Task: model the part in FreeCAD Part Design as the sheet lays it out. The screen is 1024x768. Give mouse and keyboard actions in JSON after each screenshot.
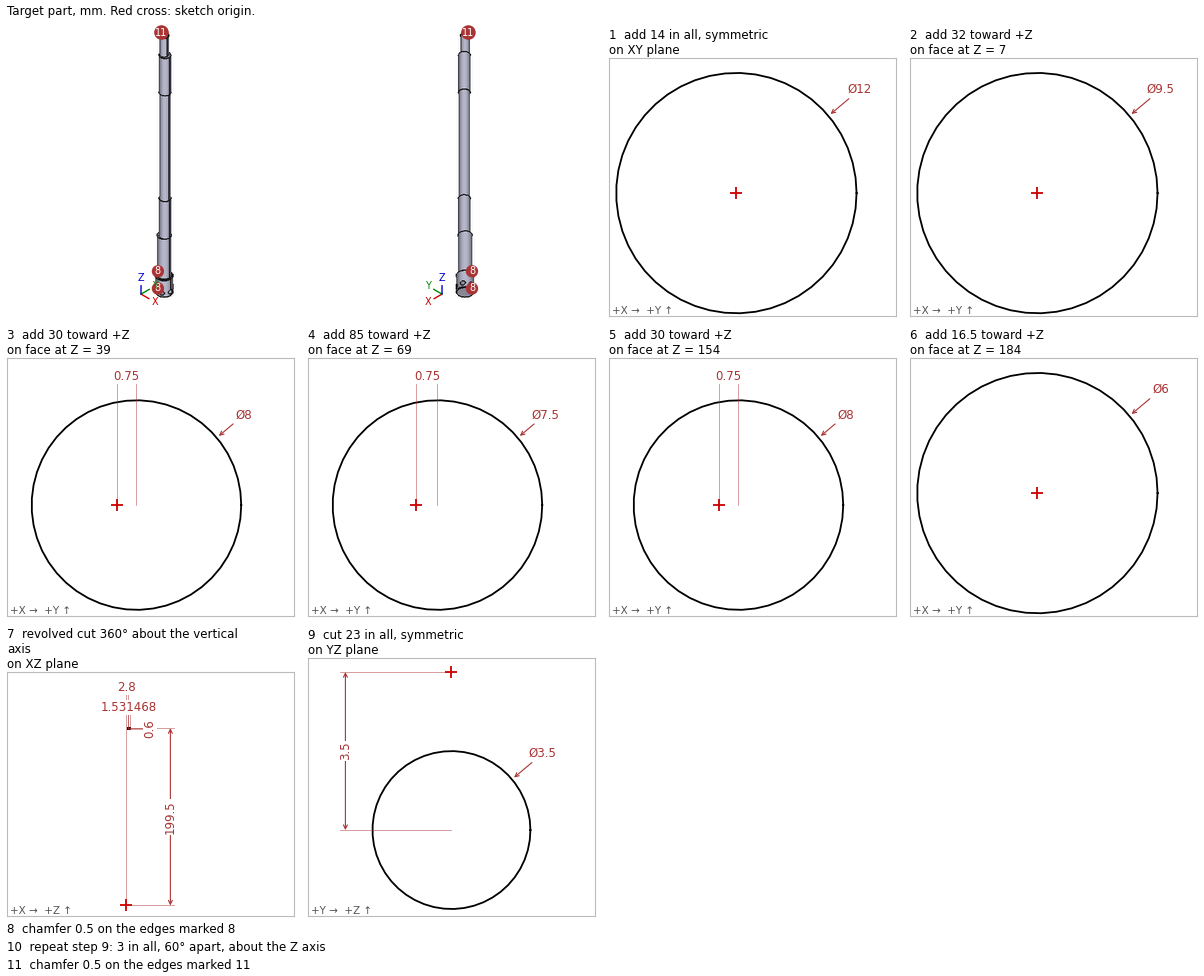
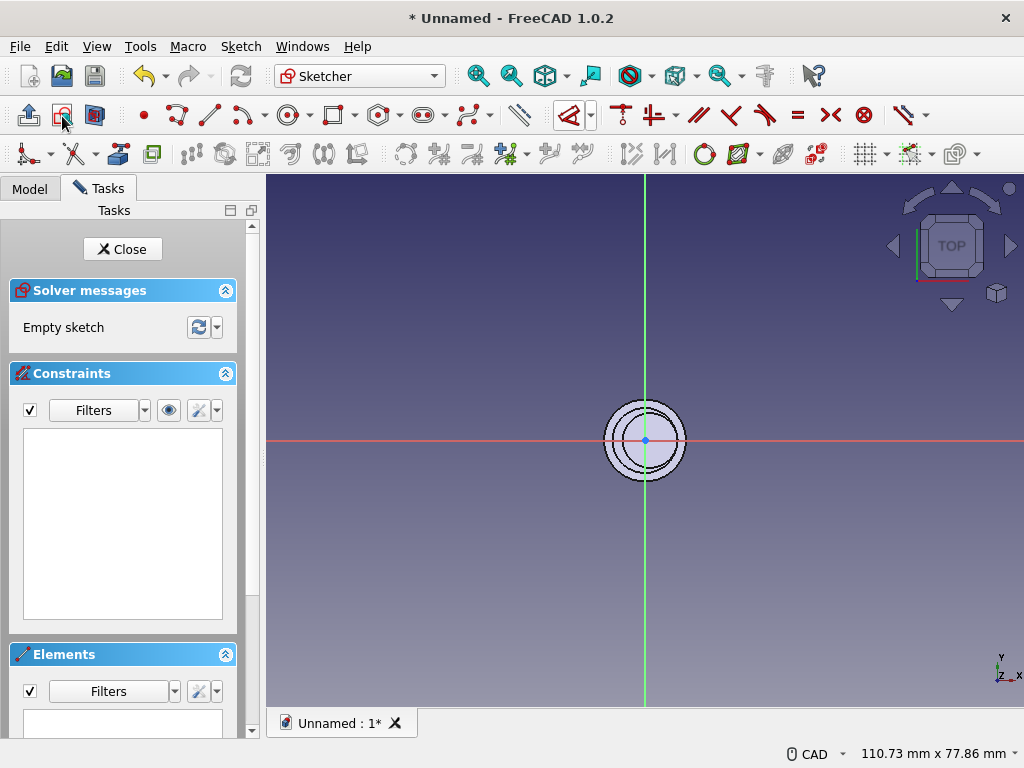
{"action": "scroll", "coordinate": [665, 440], "scroll_direction": "up", "scroll_amount": 9}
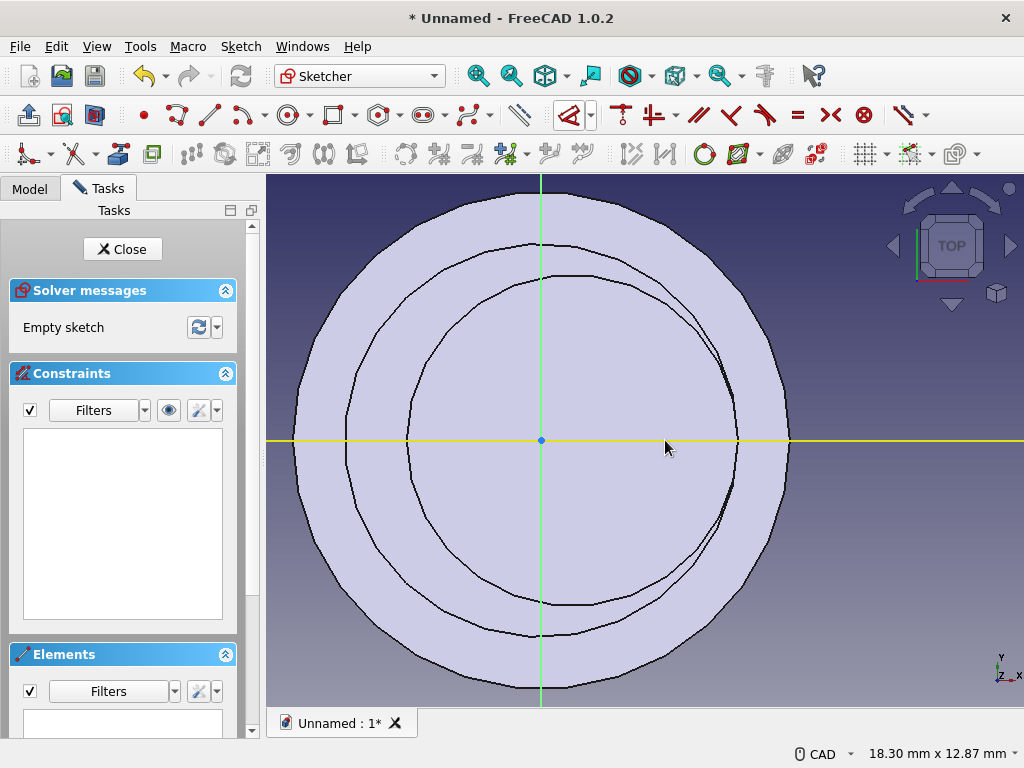
{"action": "key", "text": "g c"}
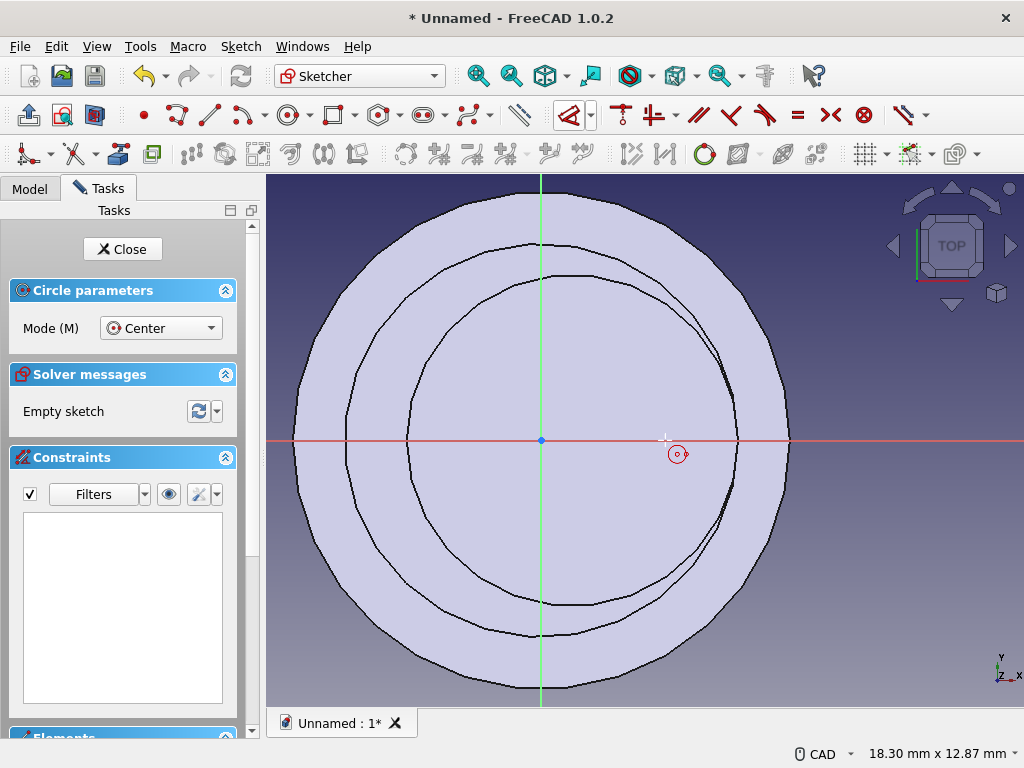
{"action": "left_click", "coordinate": [572, 440]}
{"action": "left_click", "coordinate": [682, 331]}
{"action": "key", "text": "Escape"}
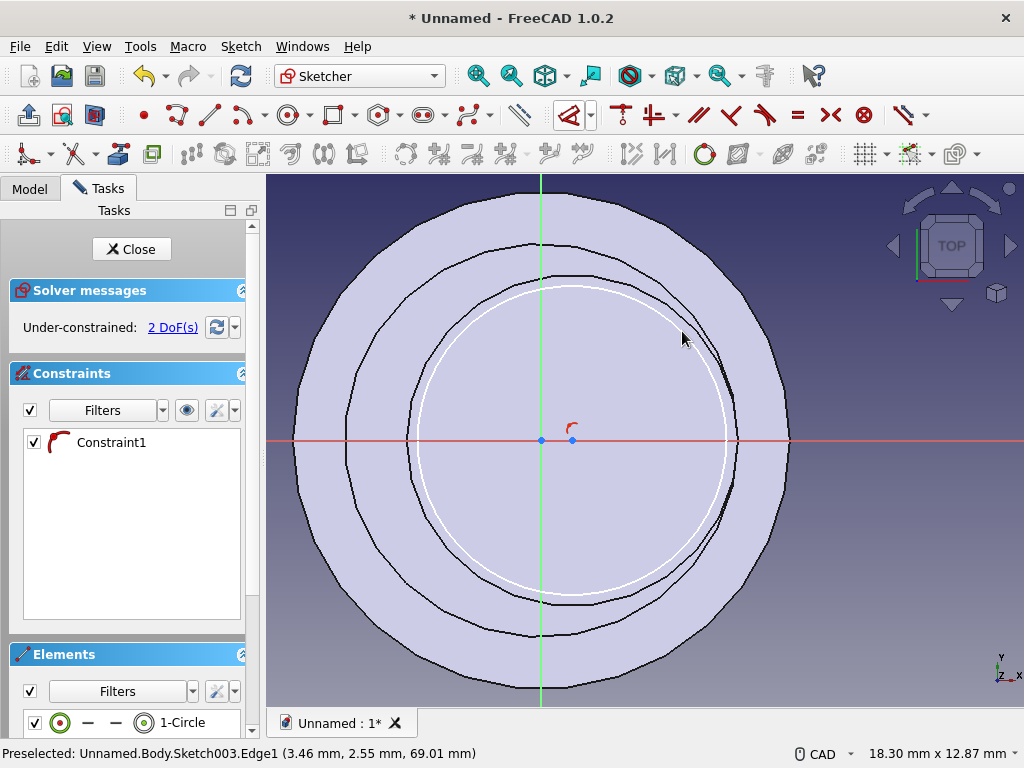
{"action": "left_click", "coordinate": [681, 331]}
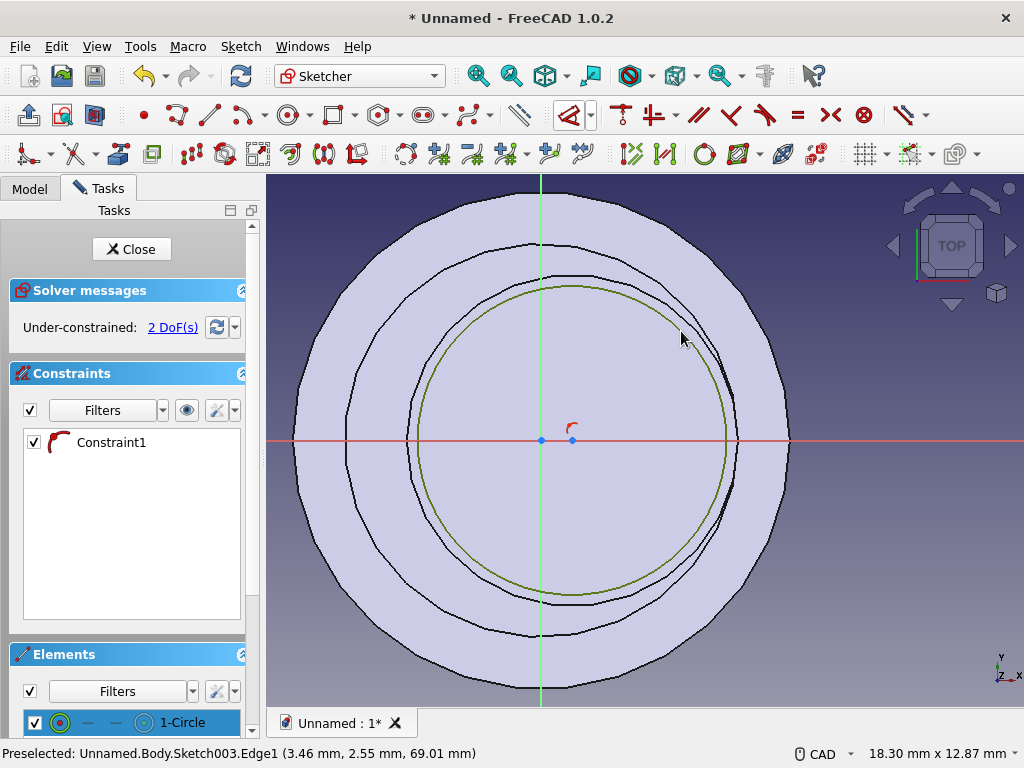
{"action": "key", "text": "k o"}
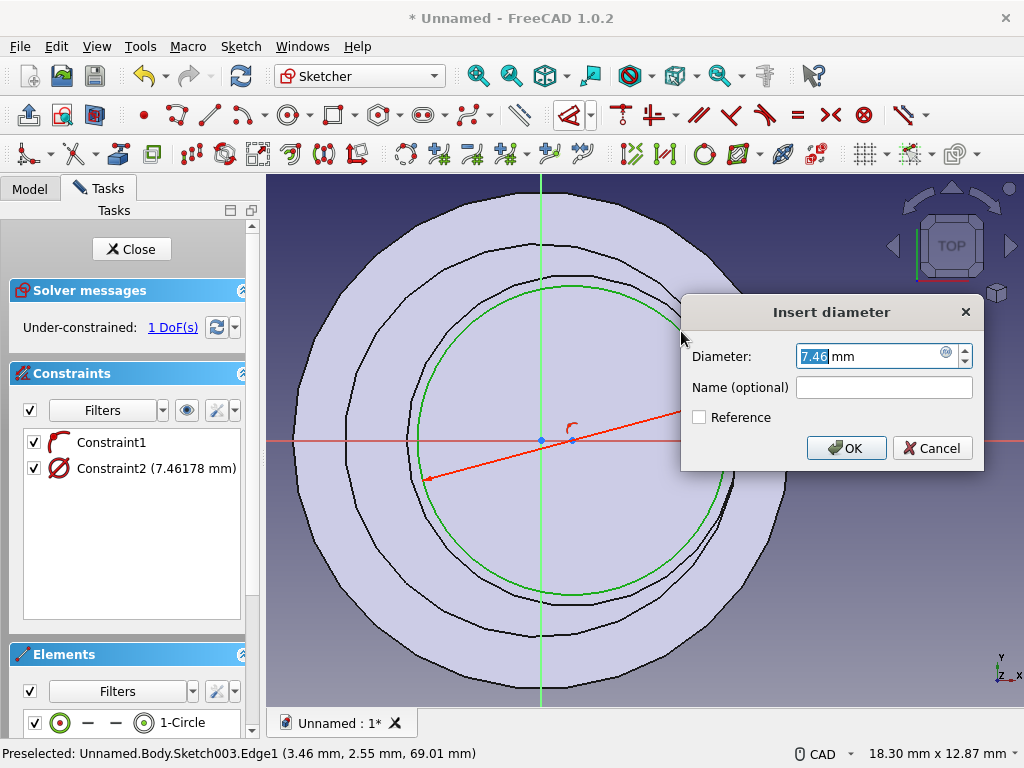
{"action": "type", "text": "7.5"}
{"action": "key", "text": "Return"}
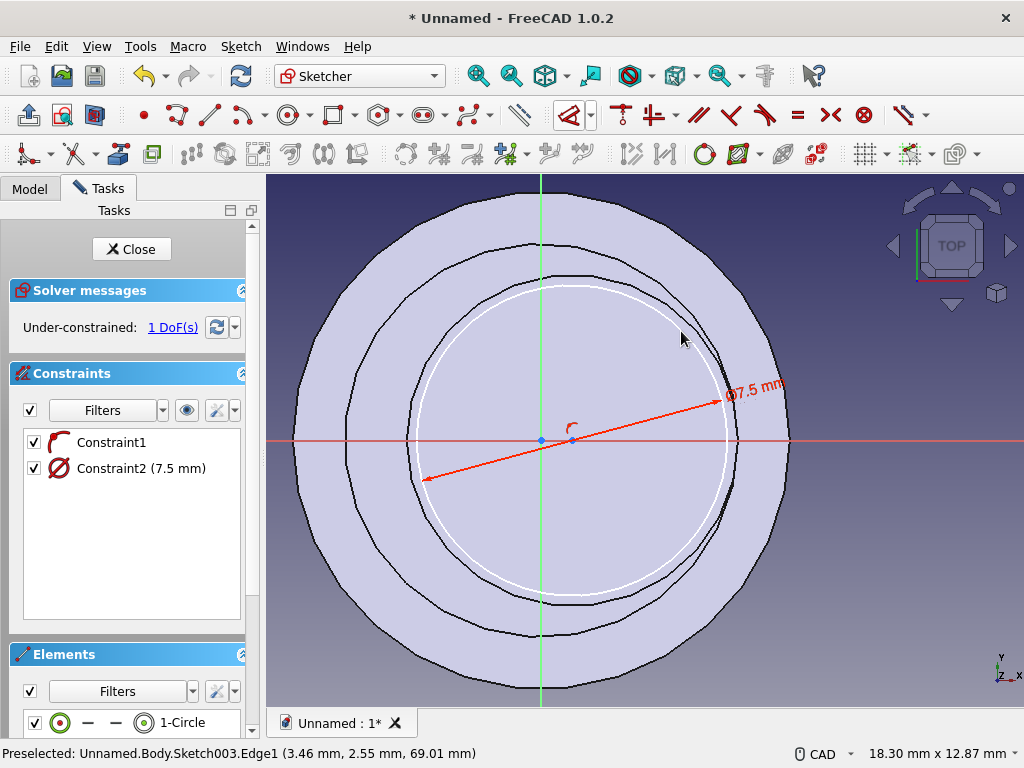
{"action": "scroll", "coordinate": [572, 440], "scroll_direction": "up", "scroll_amount": 2}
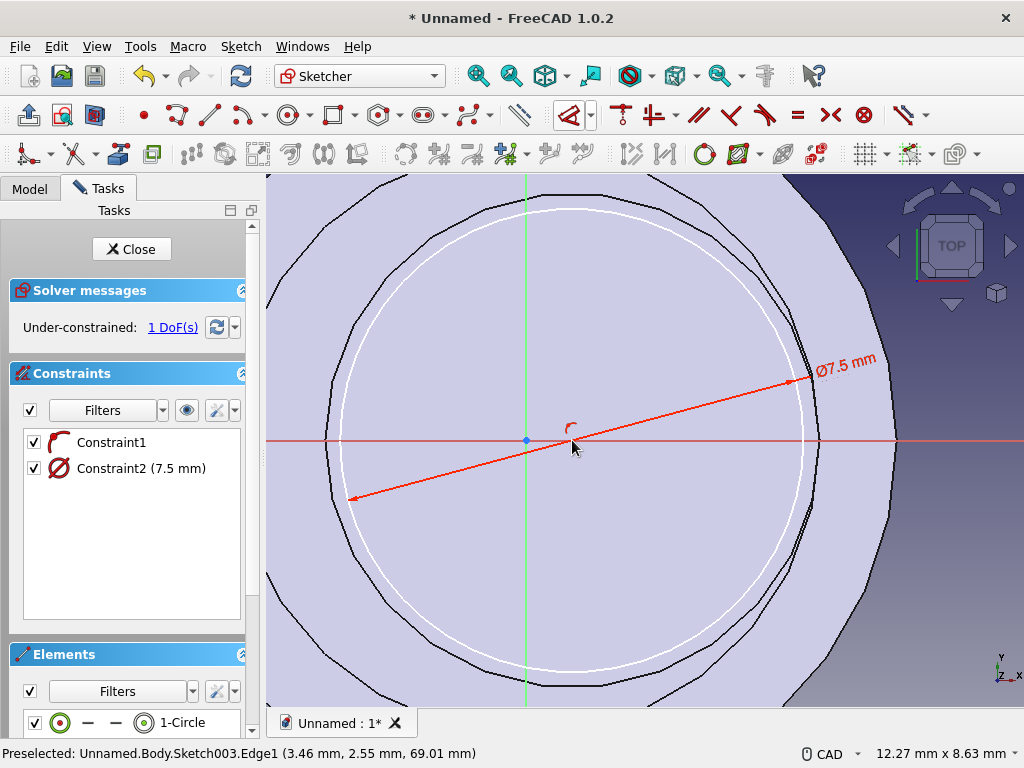
{"action": "left_click", "coordinate": [572, 440]}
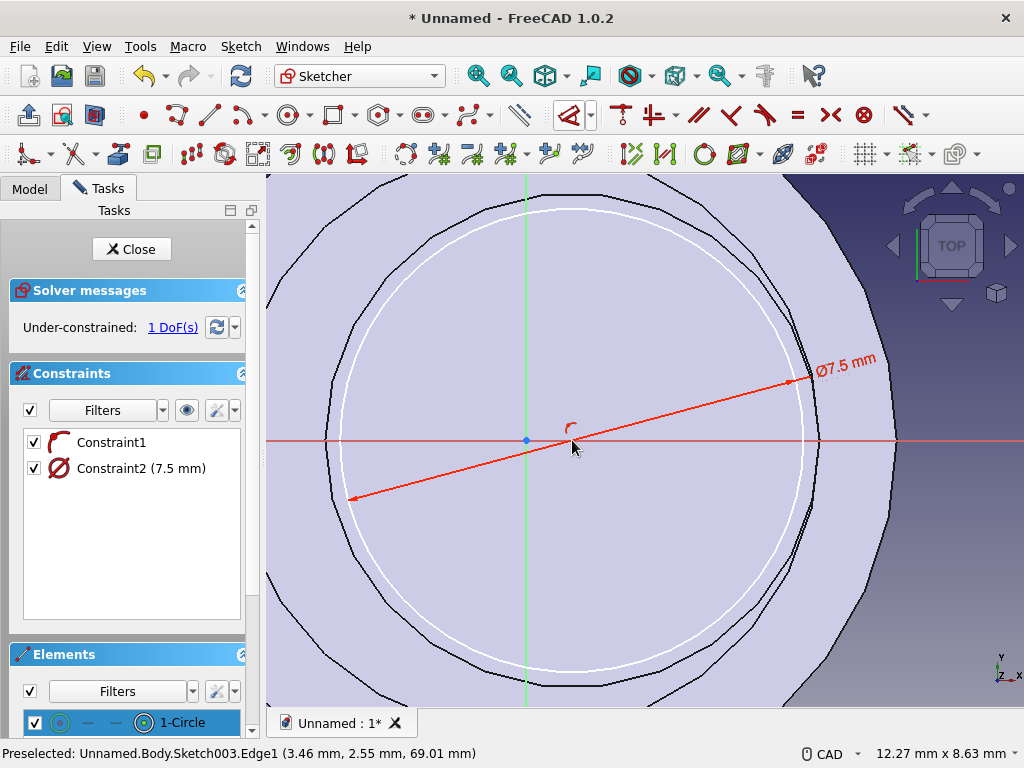
{"action": "key", "text": "l"}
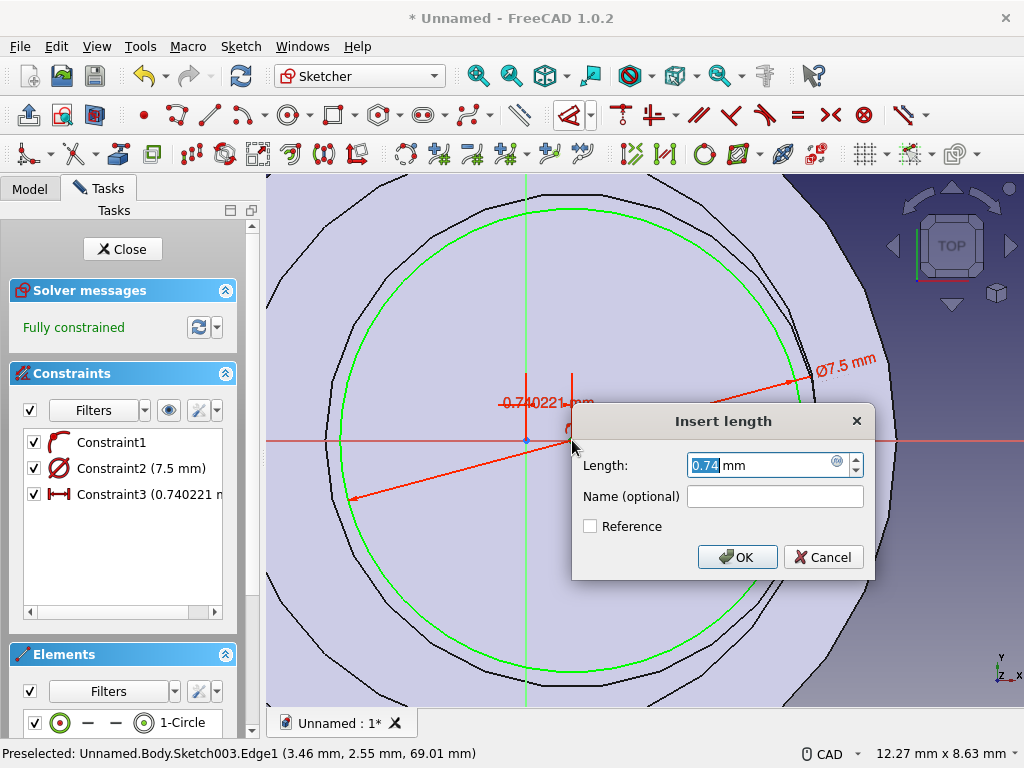
{"action": "type", "text": "0.75"}
{"action": "key", "text": "Return"}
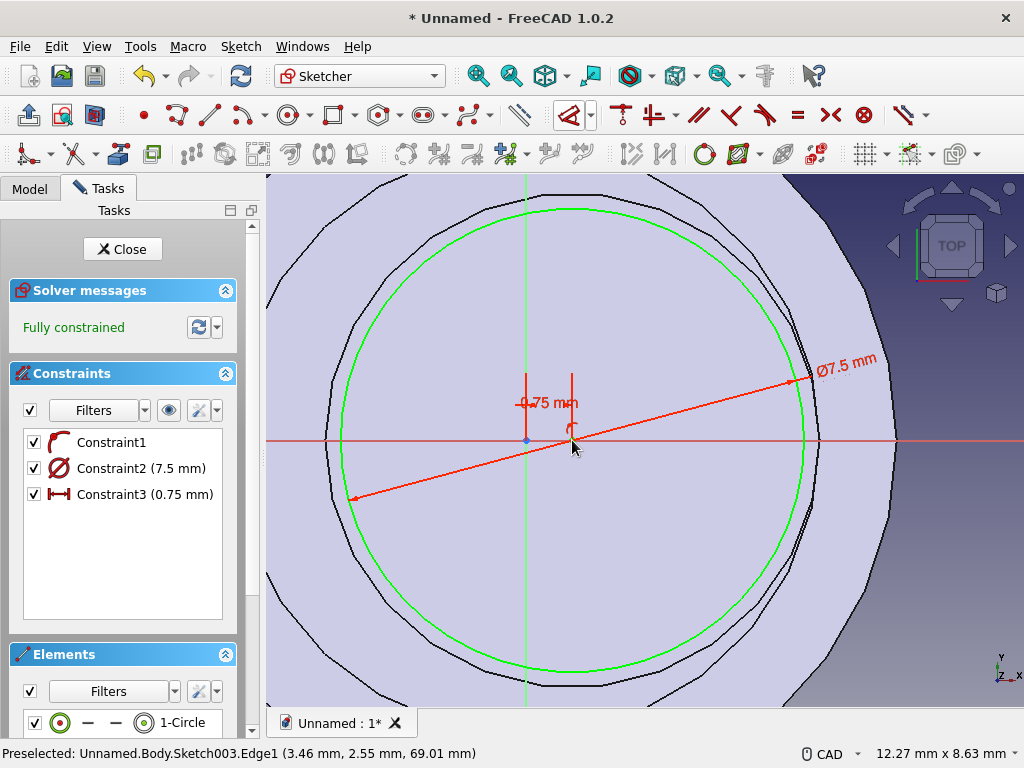
{"action": "left_click", "coordinate": [123, 249]}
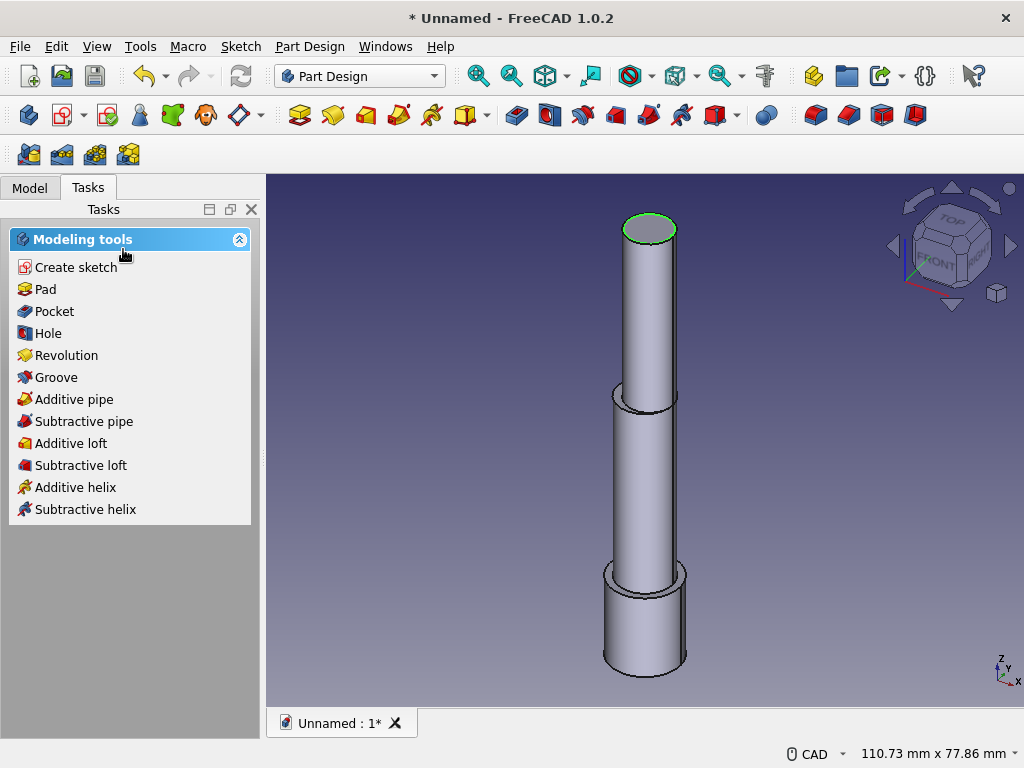
{"action": "left_click", "coordinate": [300, 116]}